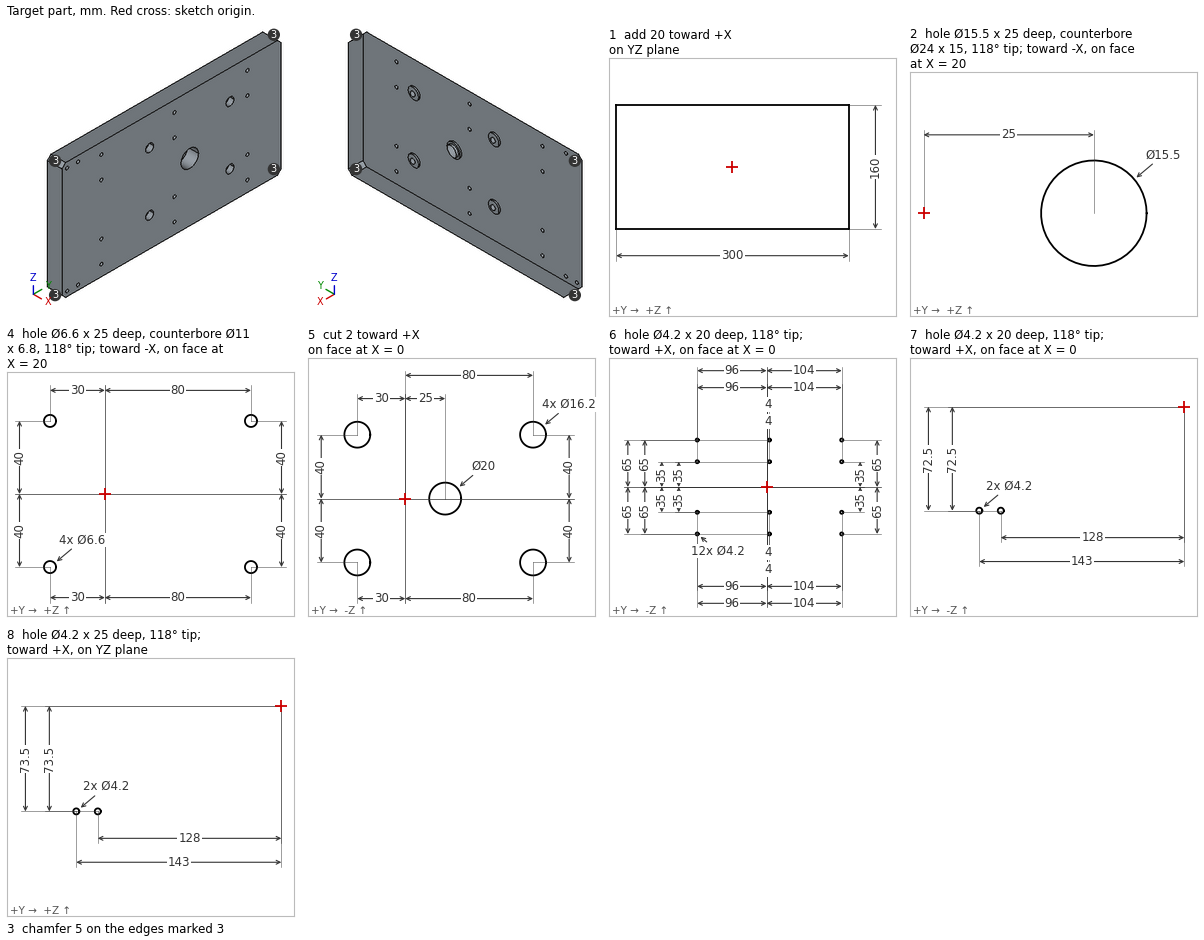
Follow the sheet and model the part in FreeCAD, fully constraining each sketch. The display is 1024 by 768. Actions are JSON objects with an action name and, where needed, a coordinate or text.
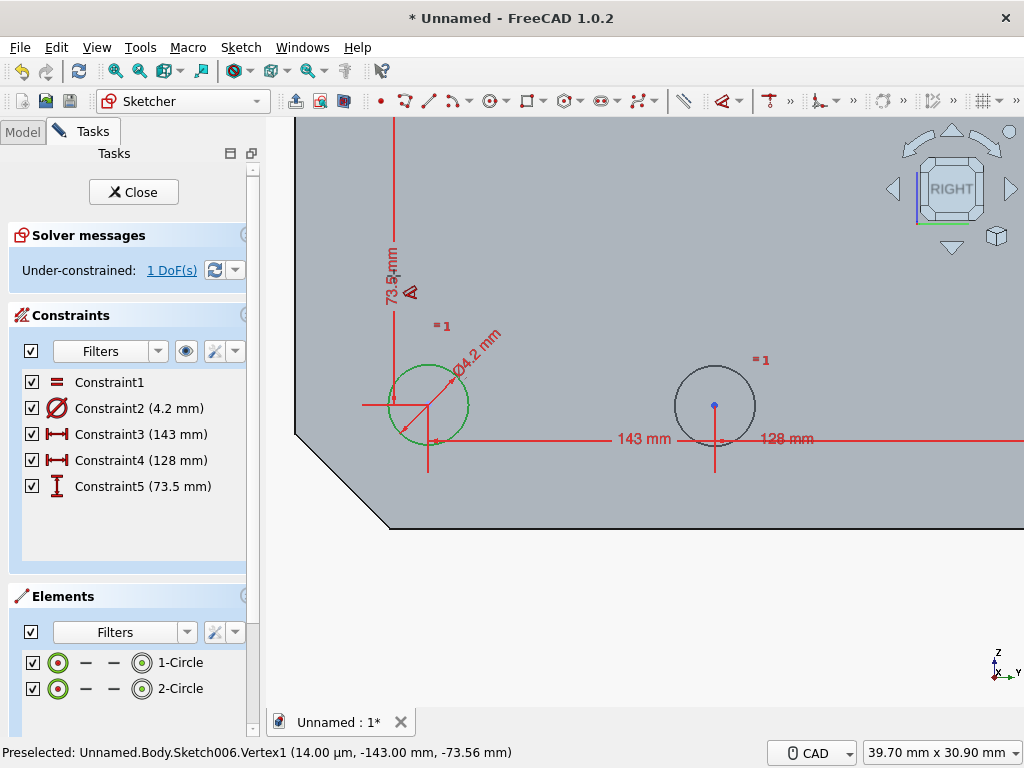
{"action": "left_click", "coordinate": [715, 406]}
{"action": "left_click", "coordinate": [681, 276]}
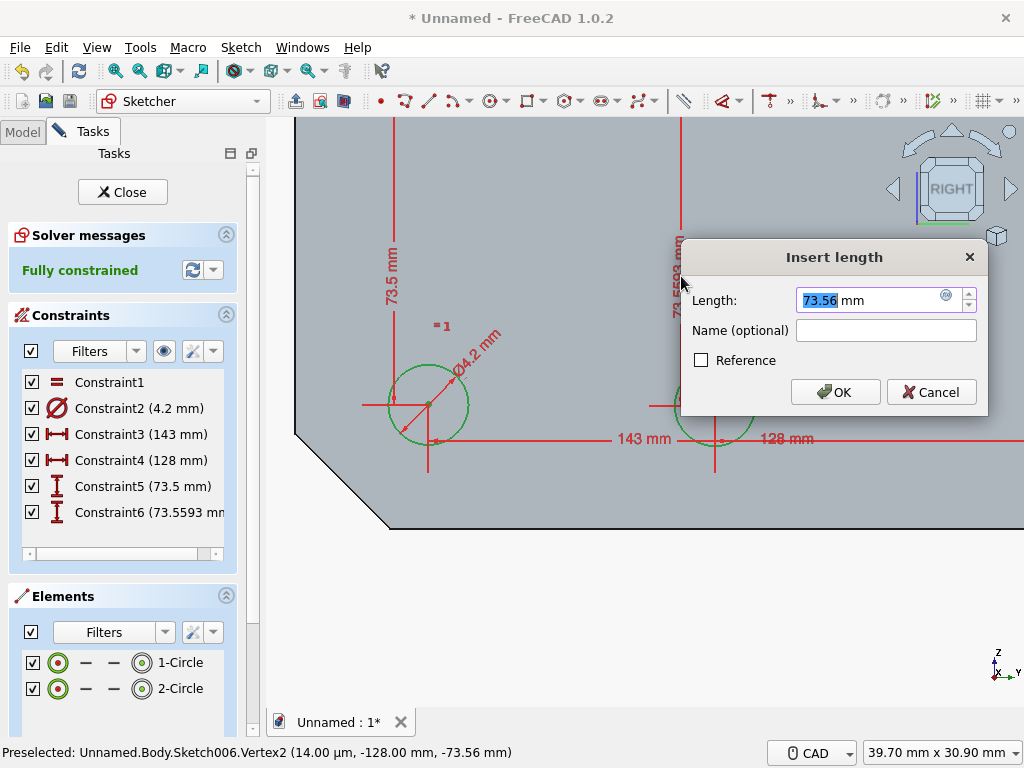
{"action": "type", "text": "73.5"}
{"action": "key", "text": "Return"}
{"action": "key", "text": "Escape"}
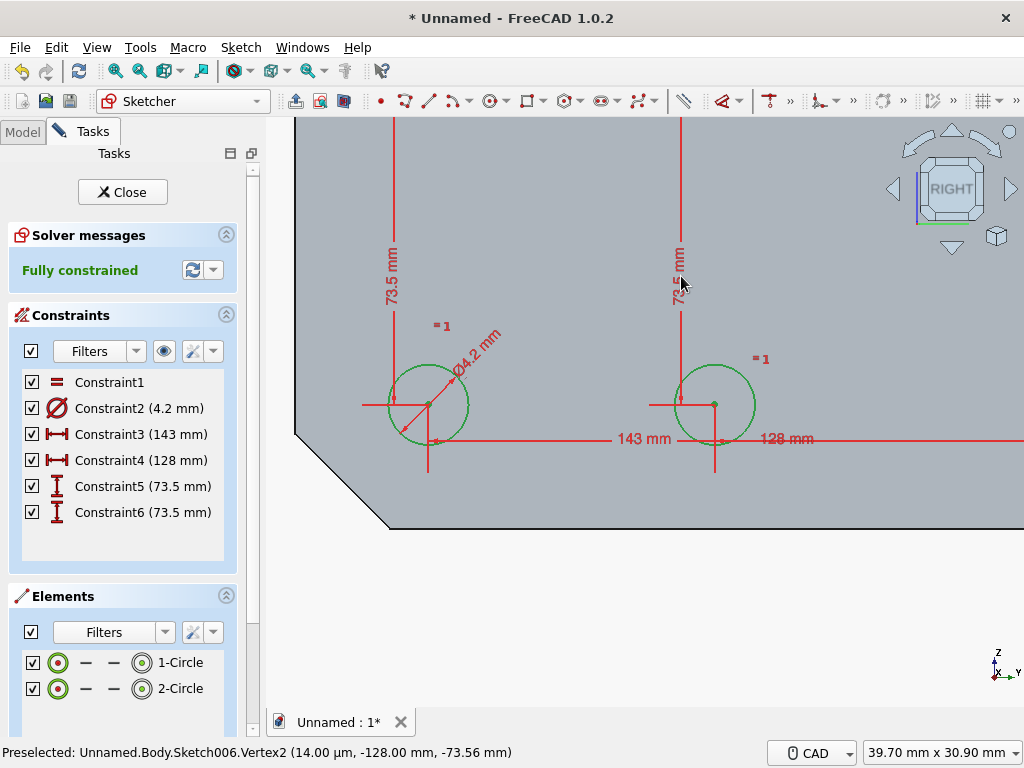
{"action": "left_click", "coordinate": [123, 192]}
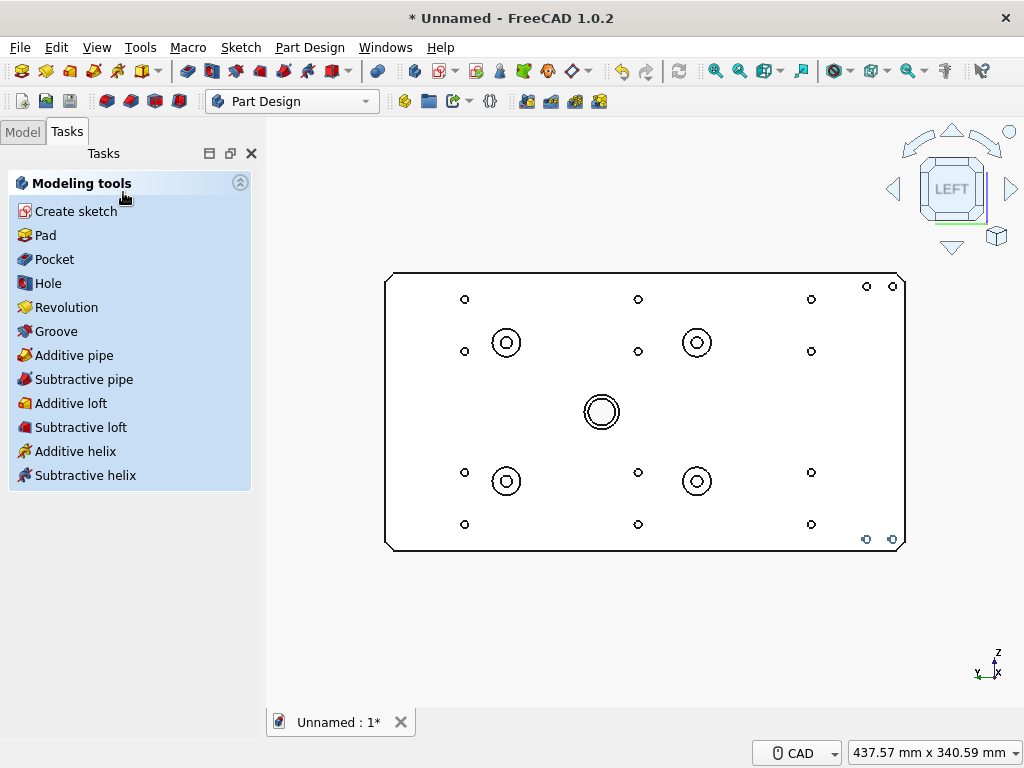
{"action": "left_click", "coordinate": [212, 72]}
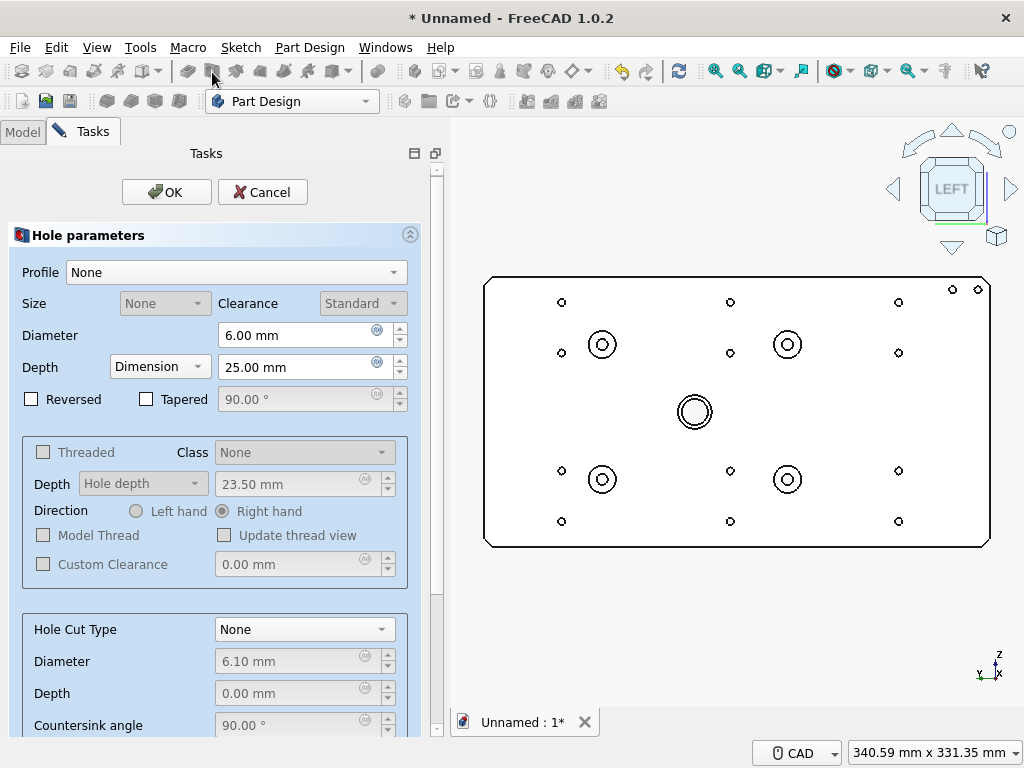
{"action": "triple_click", "coordinate": [305, 335]}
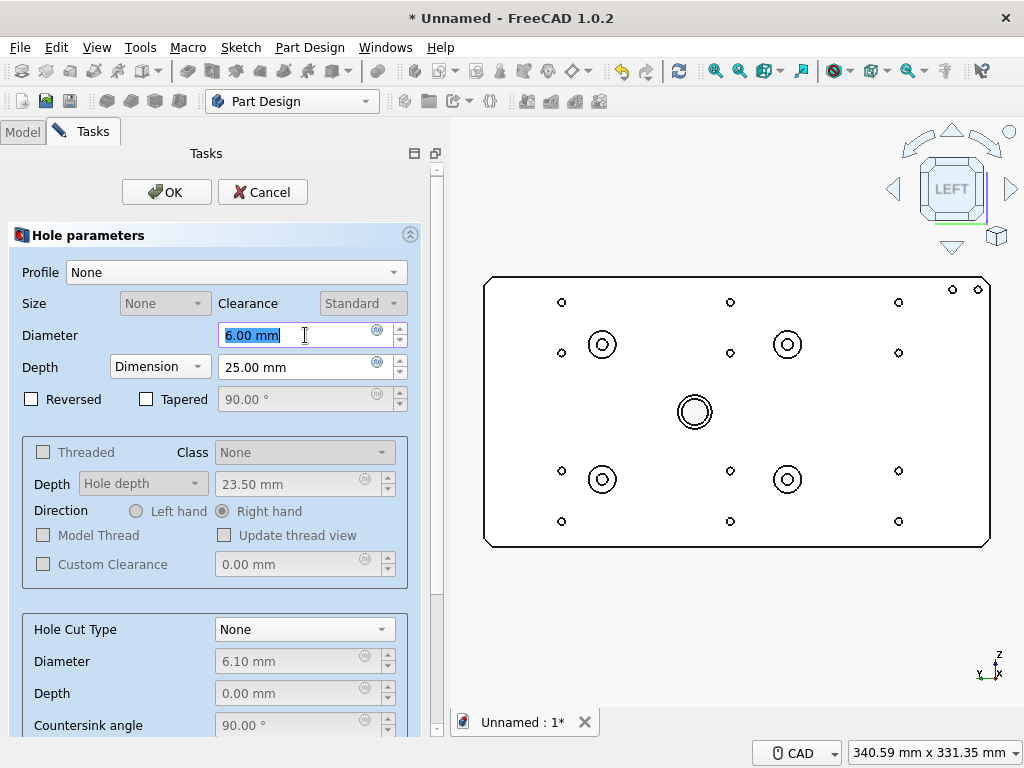
{"action": "type", "text": "4.2"}
{"action": "key", "text": "Tab"}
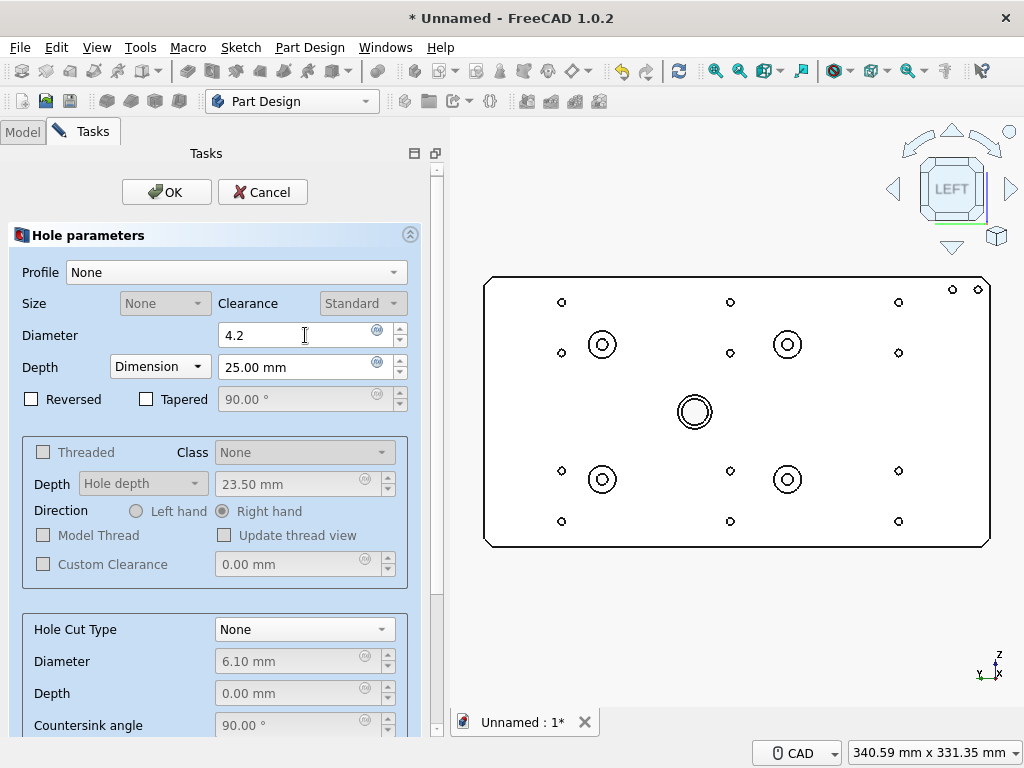
{"action": "triple_click", "coordinate": [305, 367]}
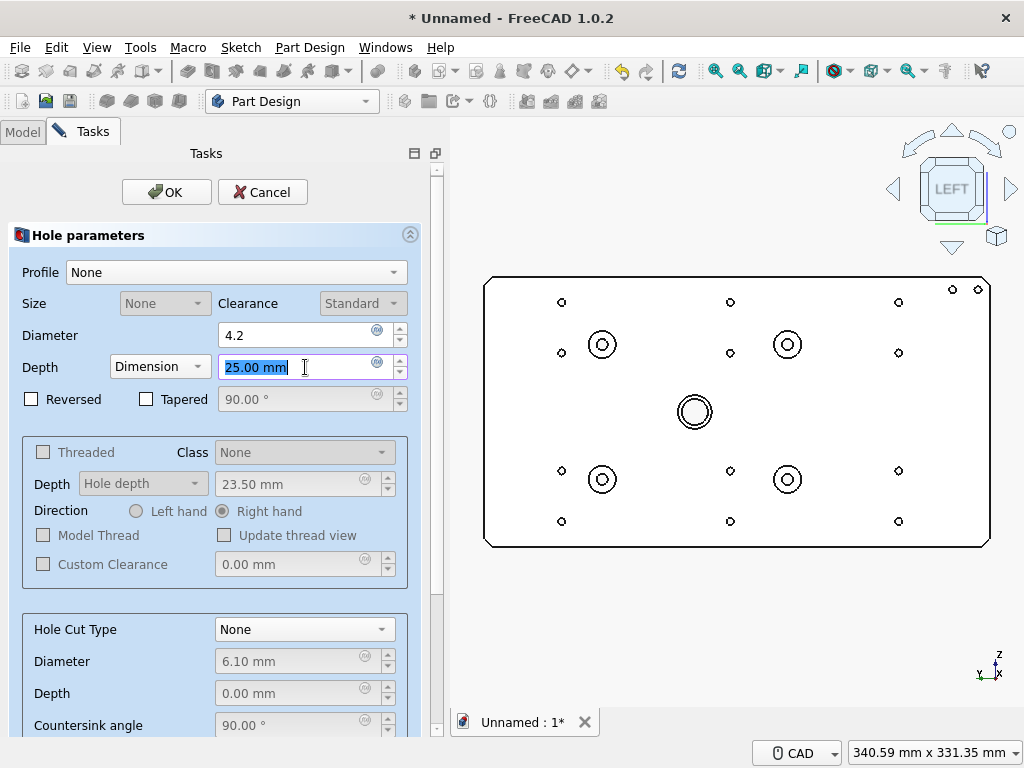
{"action": "type", "text": "25"}
{"action": "key", "text": "Tab"}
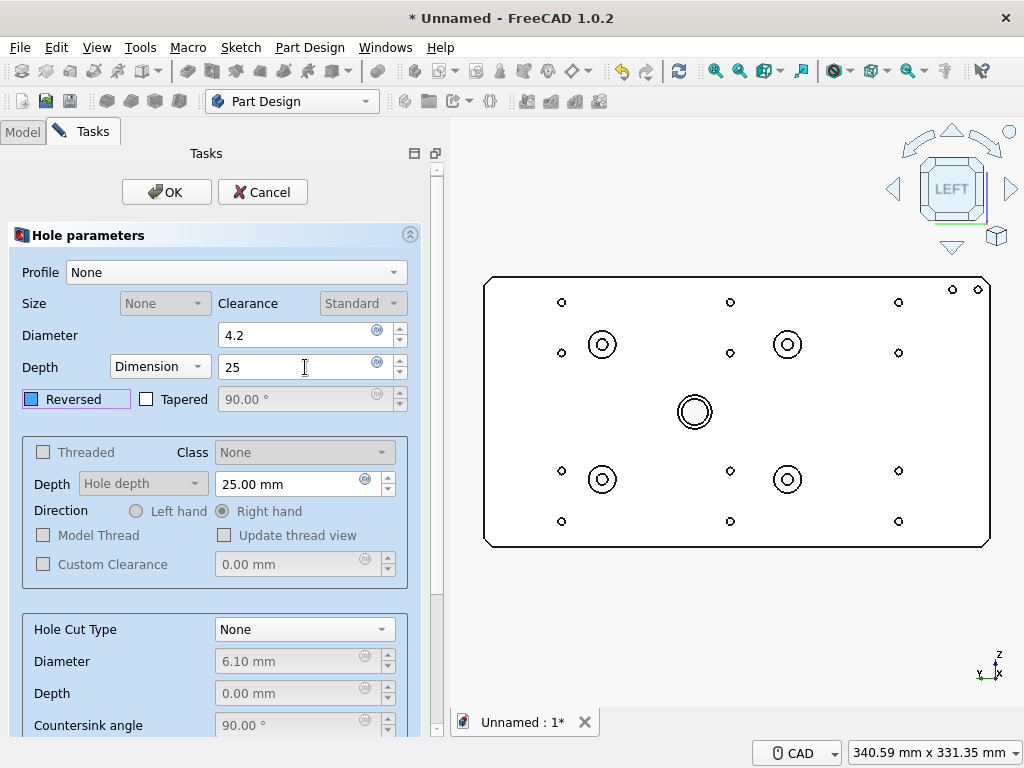
{"action": "left_click", "coordinate": [30, 399]}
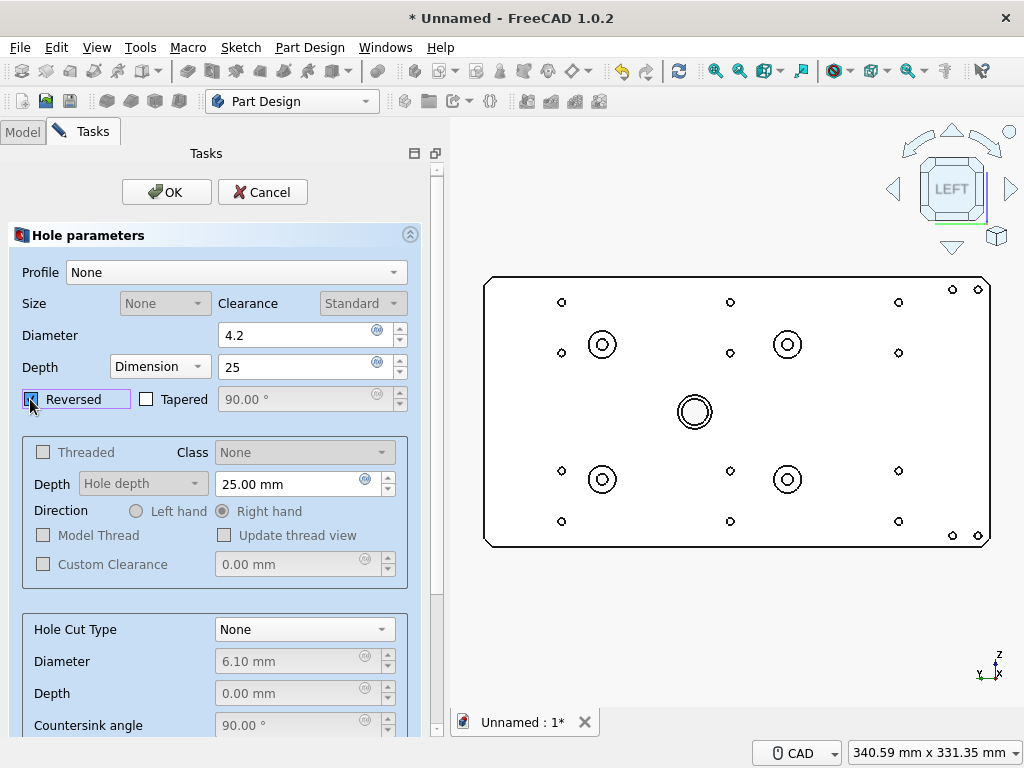
{"action": "left_click", "coordinate": [167, 192]}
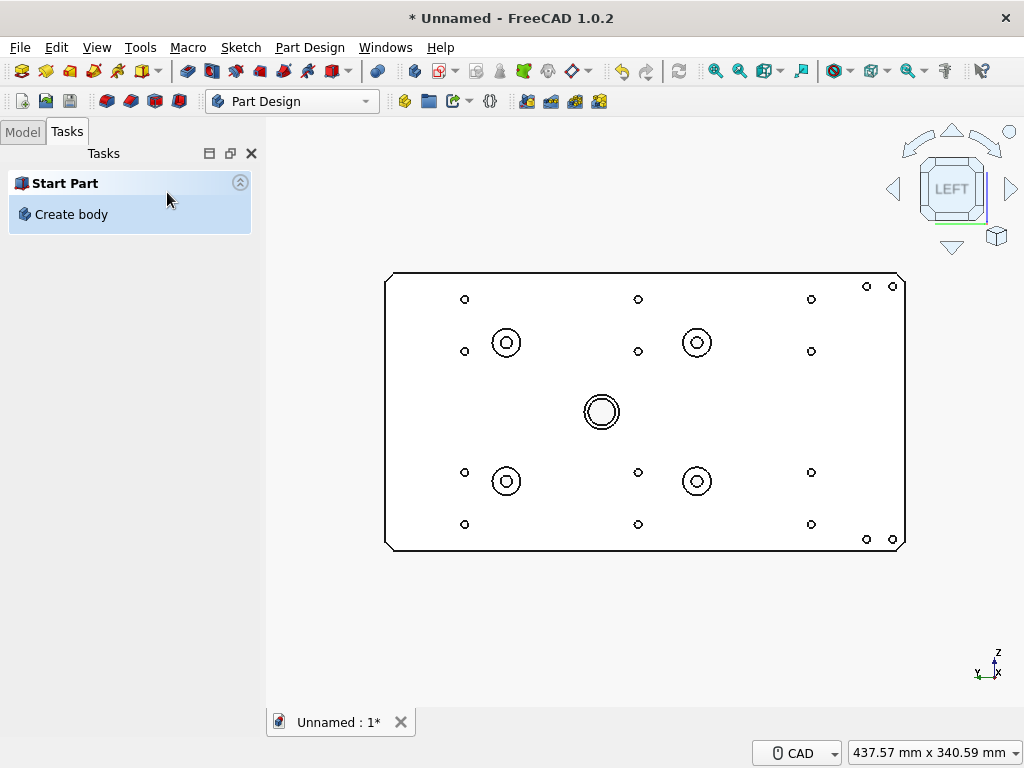
{"action": "key", "text": "0"}